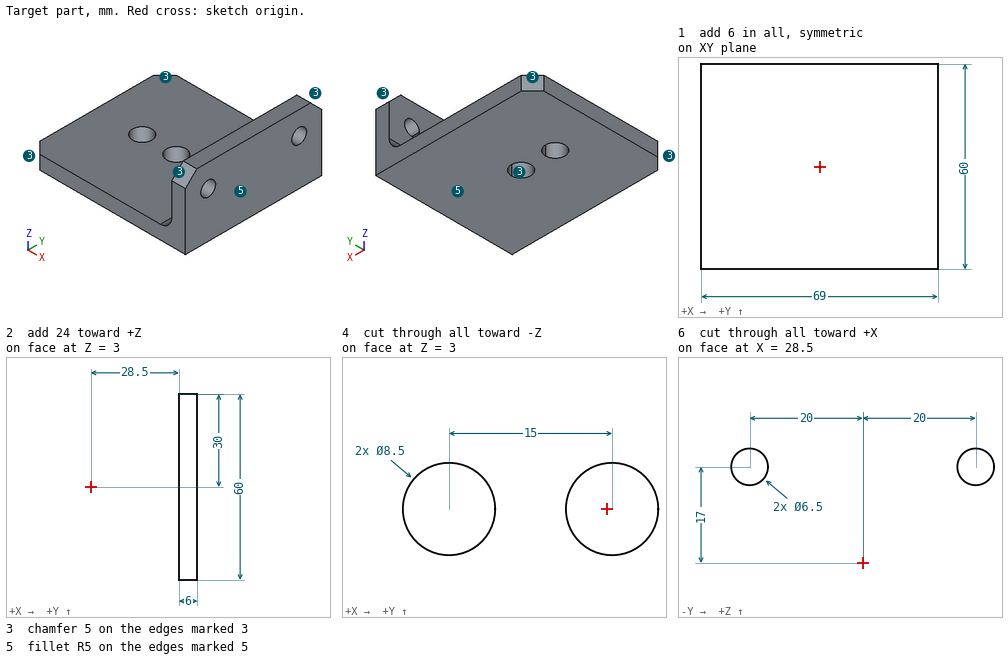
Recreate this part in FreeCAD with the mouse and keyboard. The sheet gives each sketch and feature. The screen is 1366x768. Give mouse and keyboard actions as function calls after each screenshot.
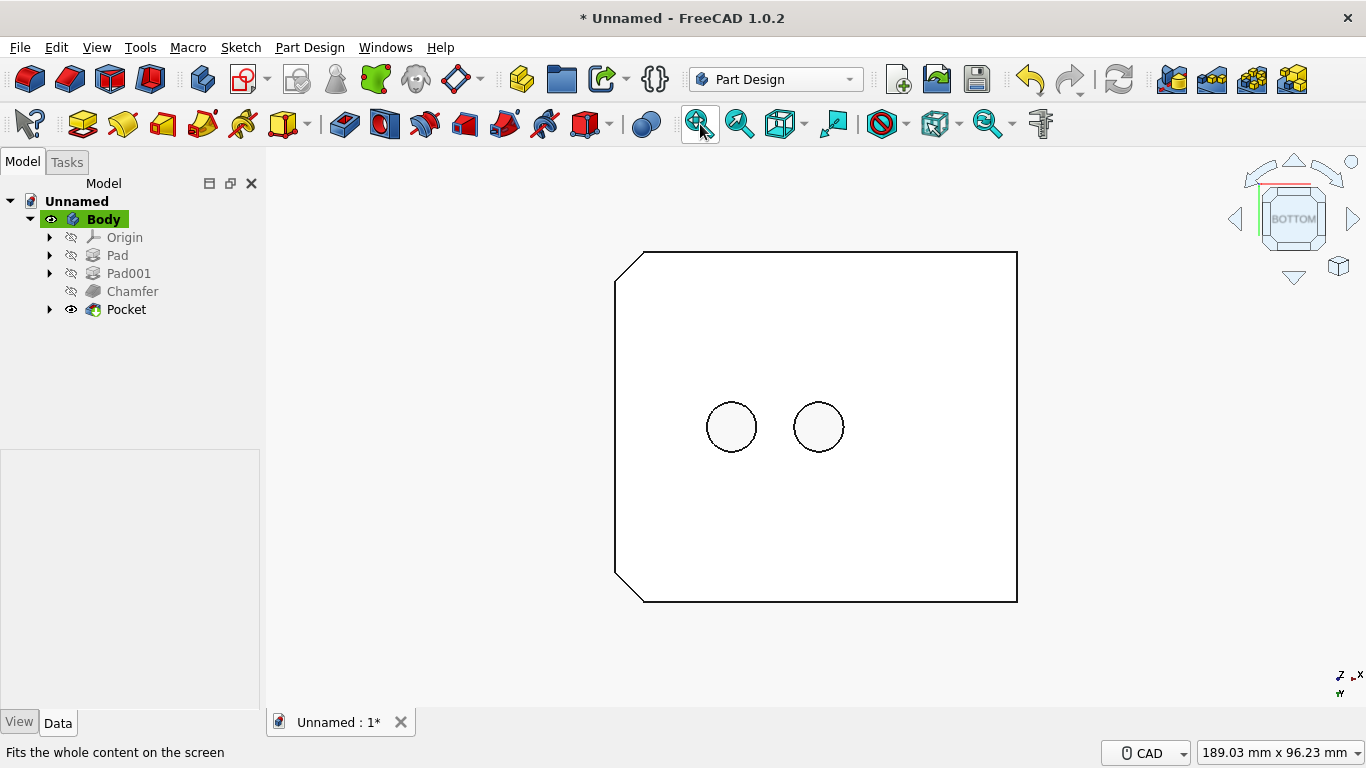
key(4)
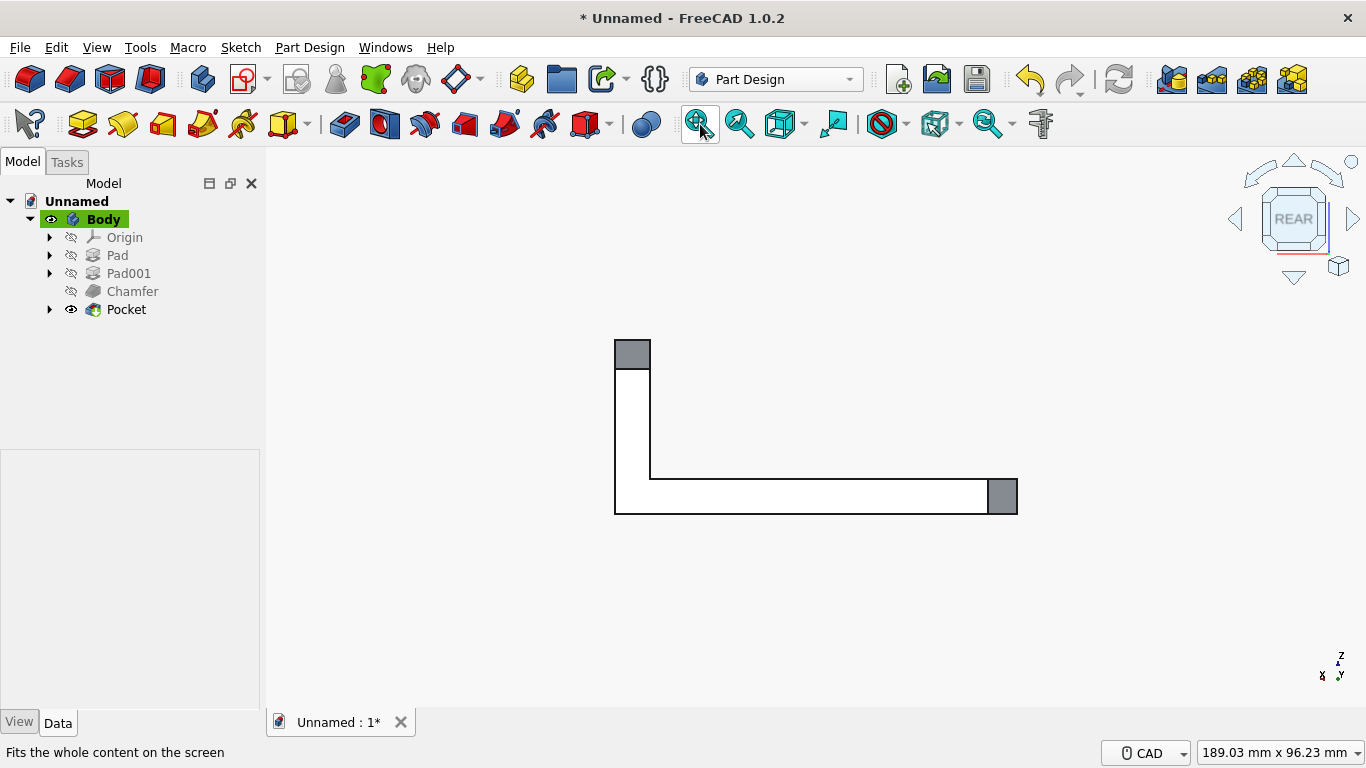
key(v)
key(f)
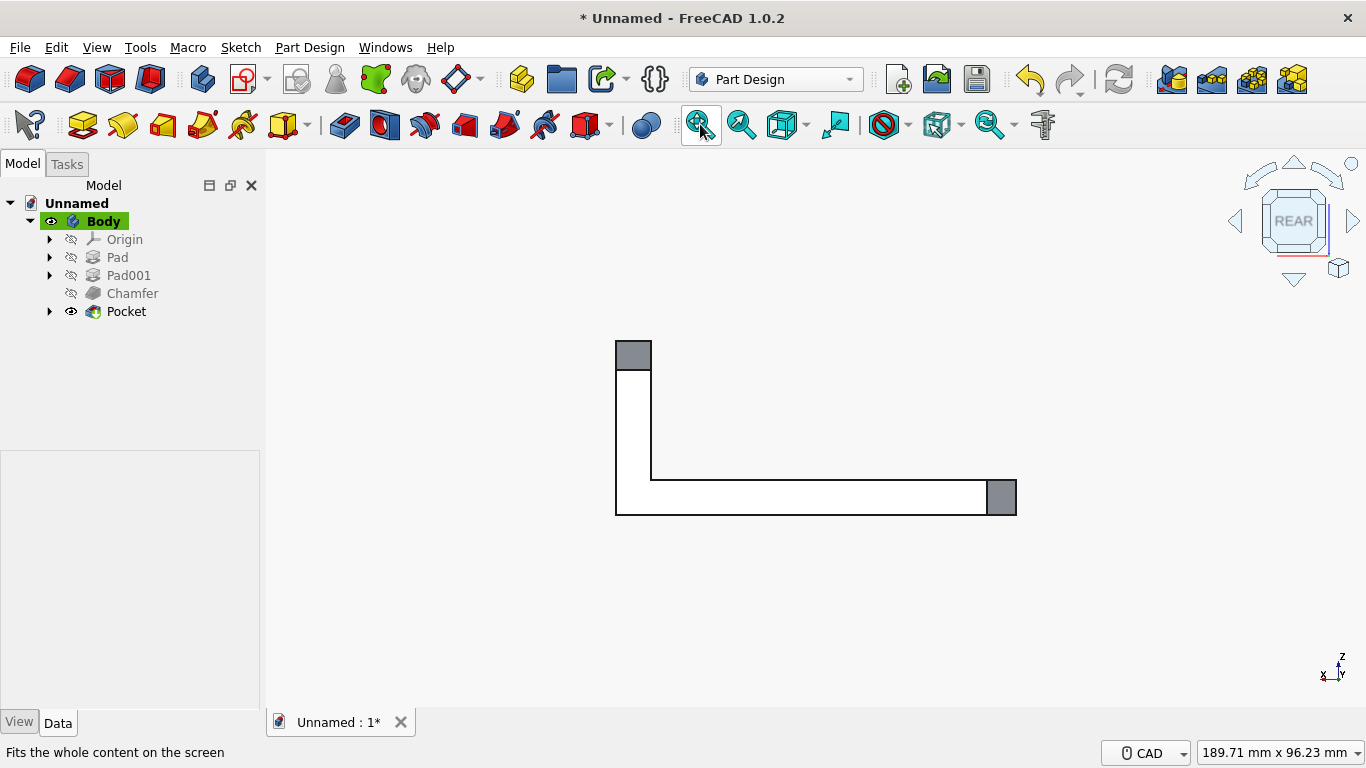
key(6)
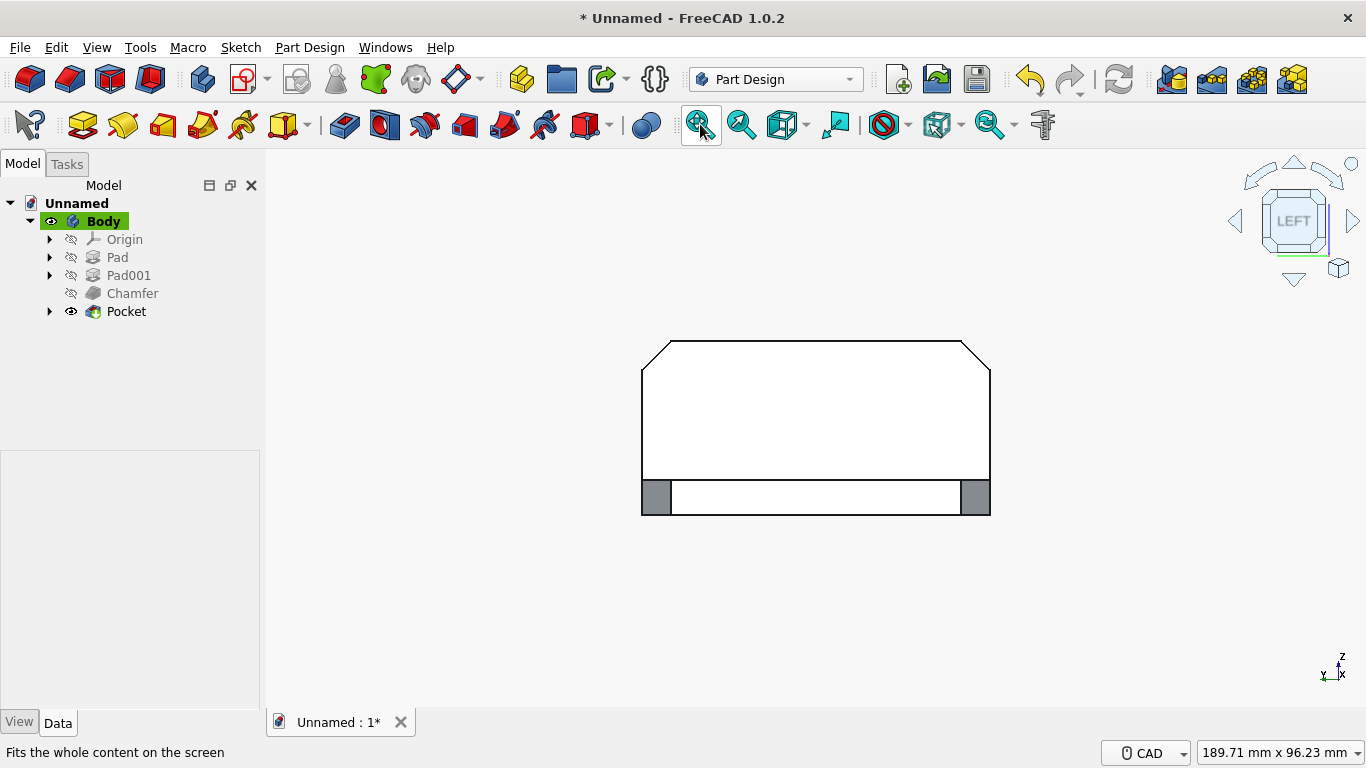
click(702, 126)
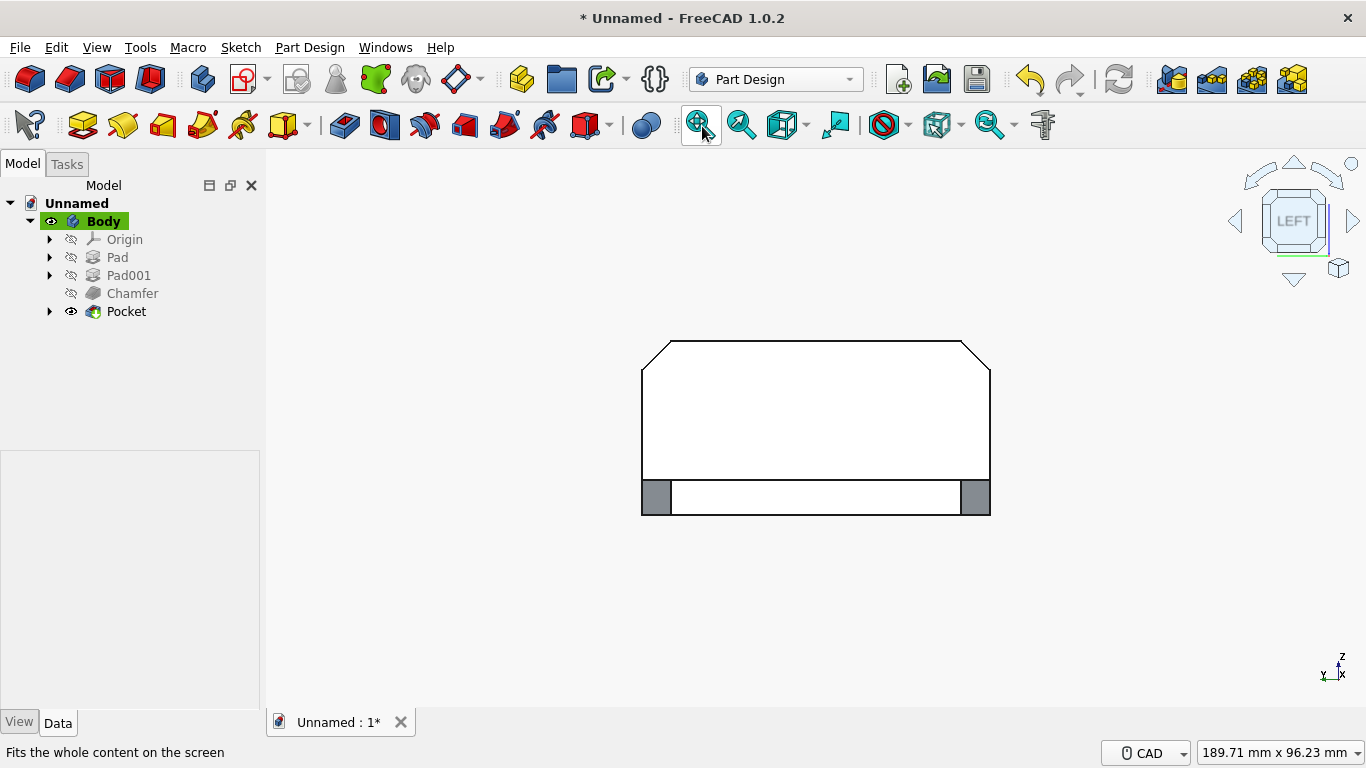
key(v)
key(3)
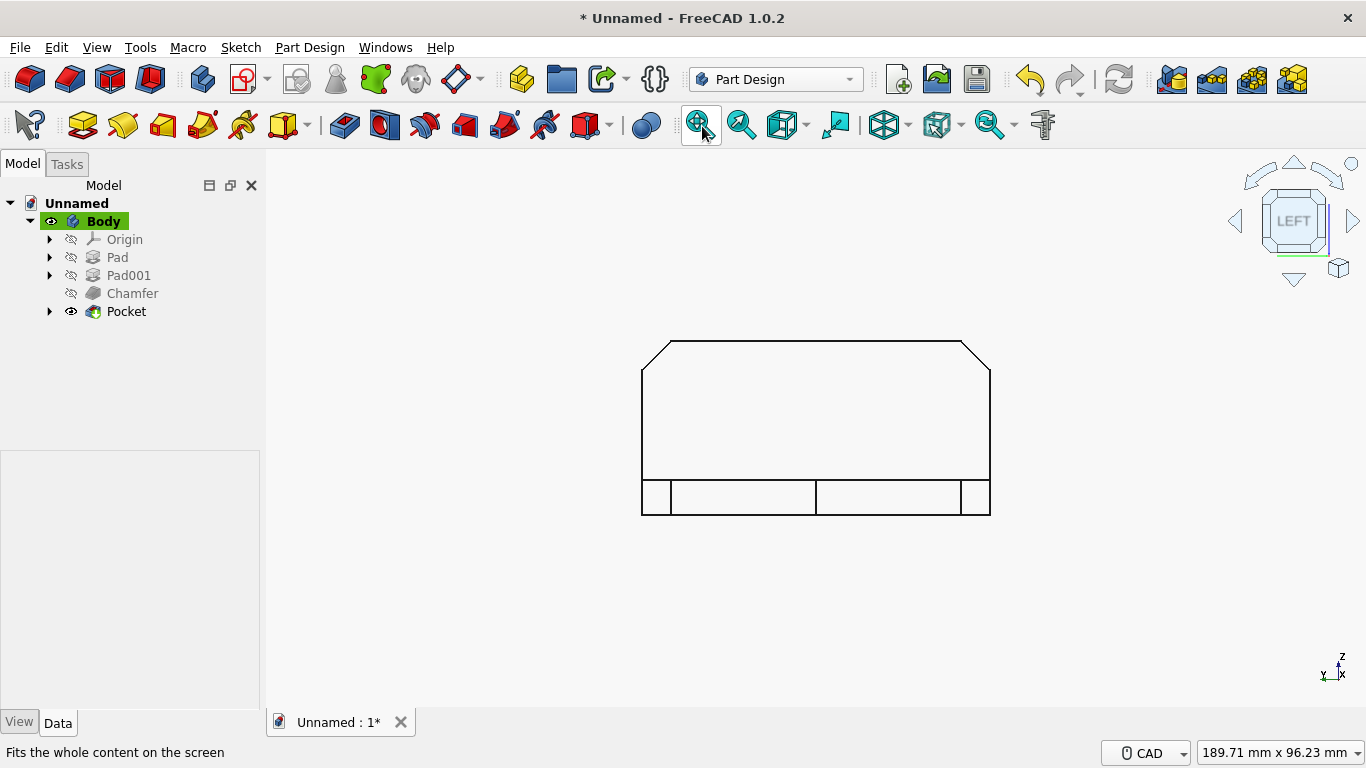
key(0)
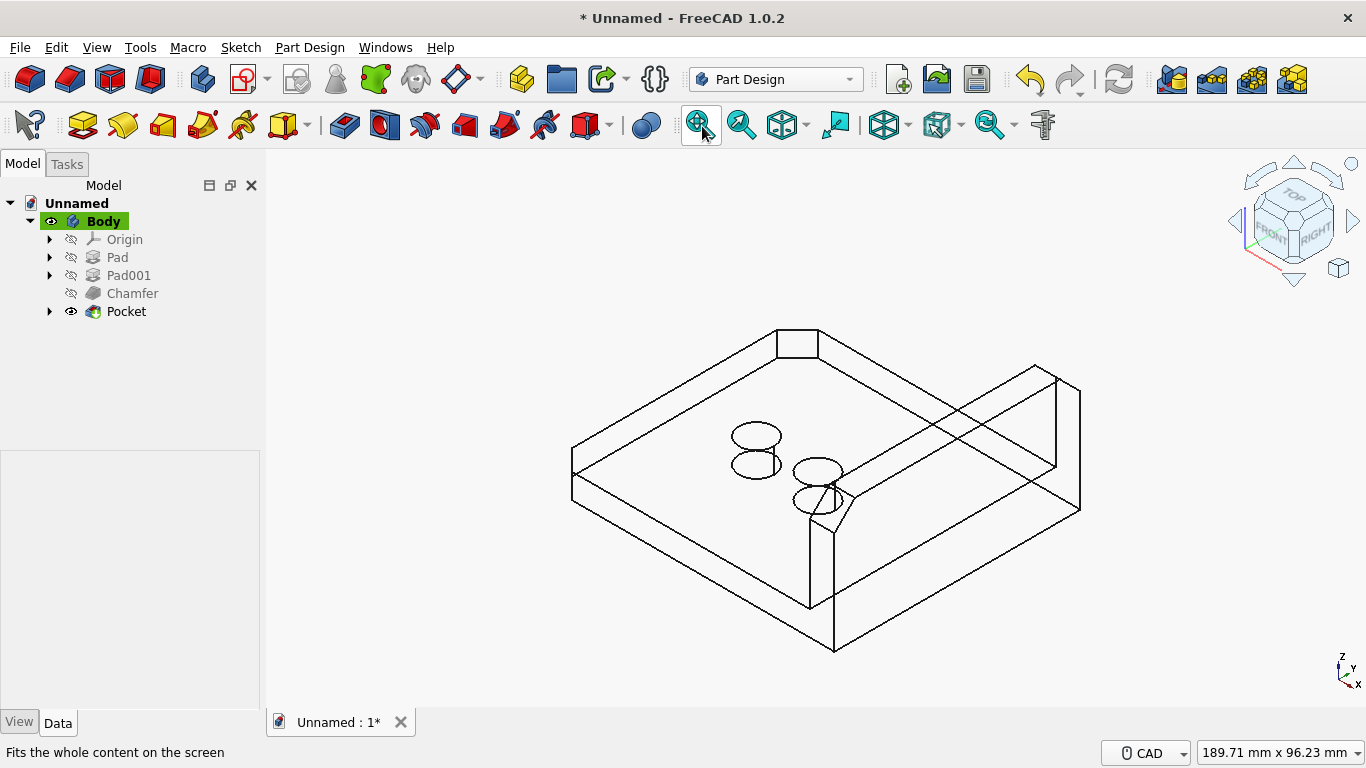
click(933, 537)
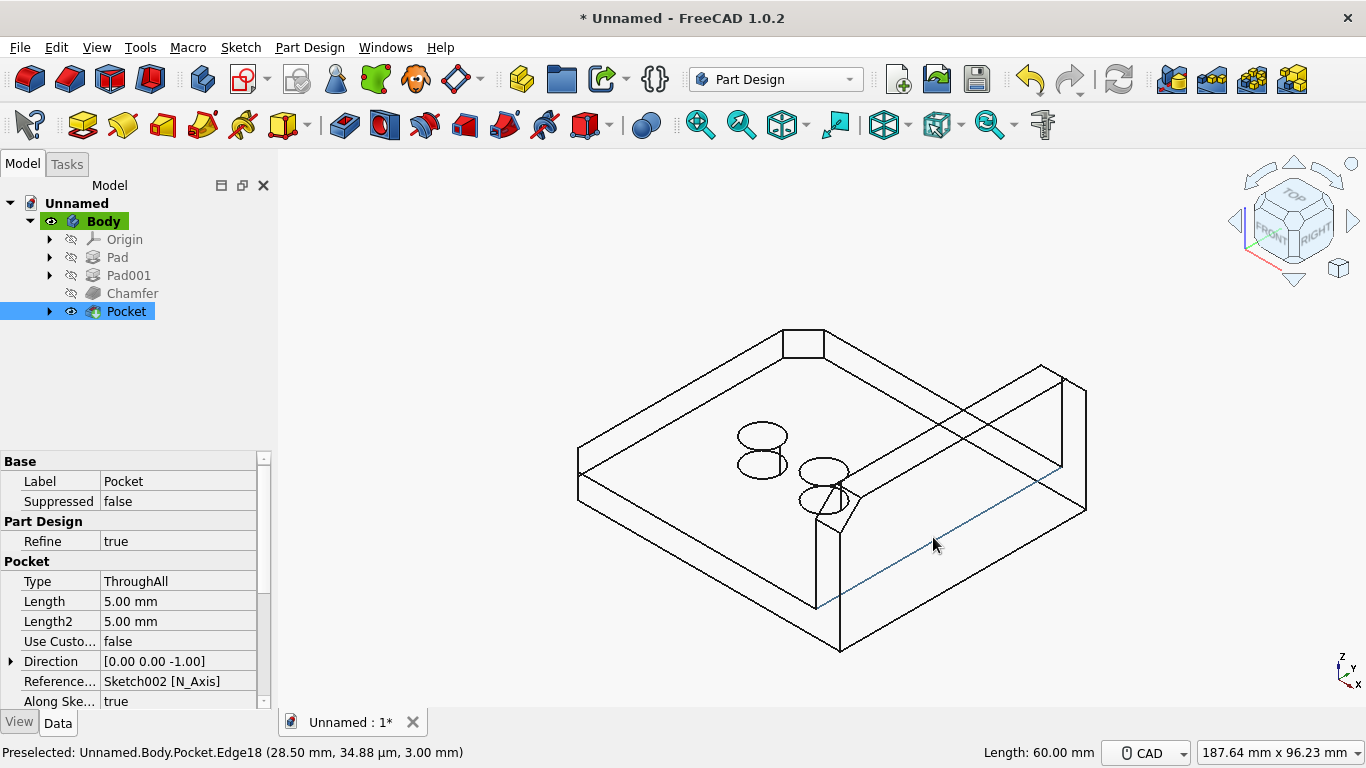
key(v)
key(1)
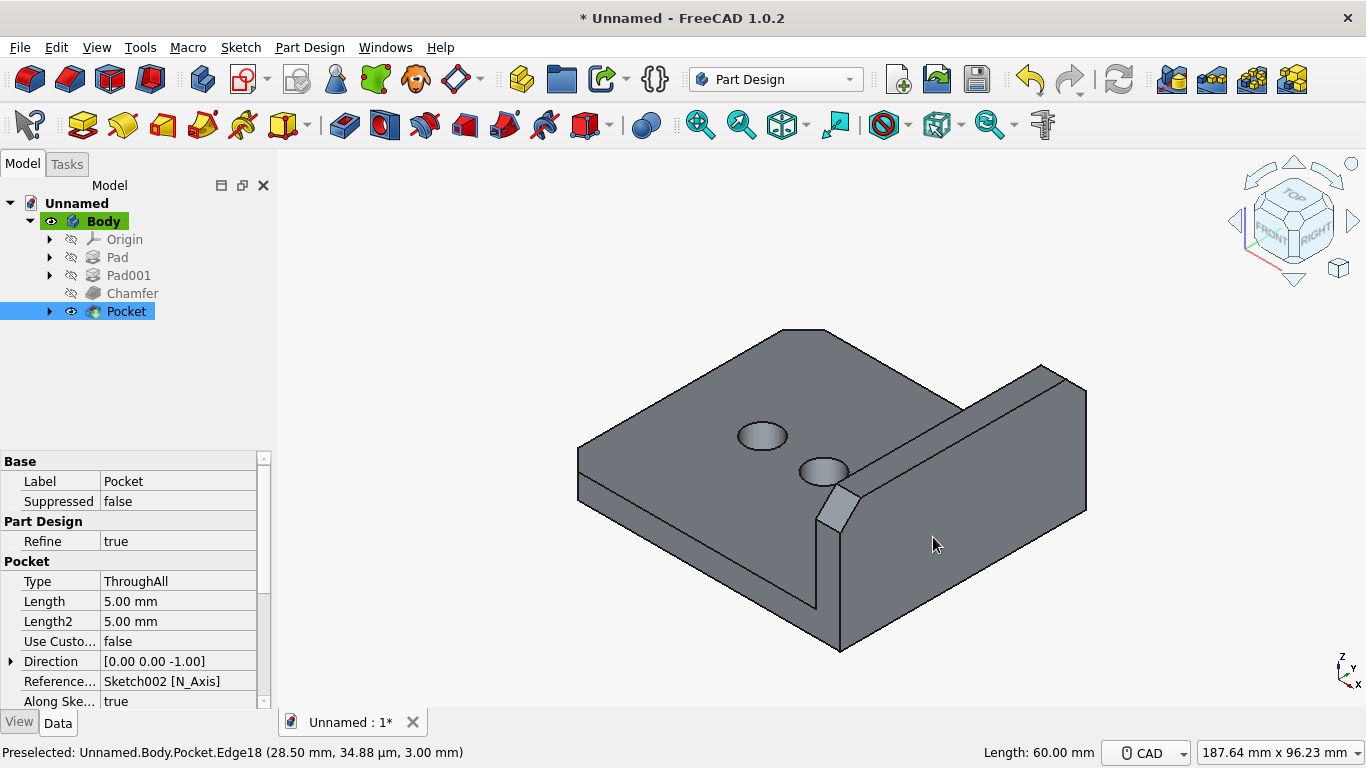
click(30, 80)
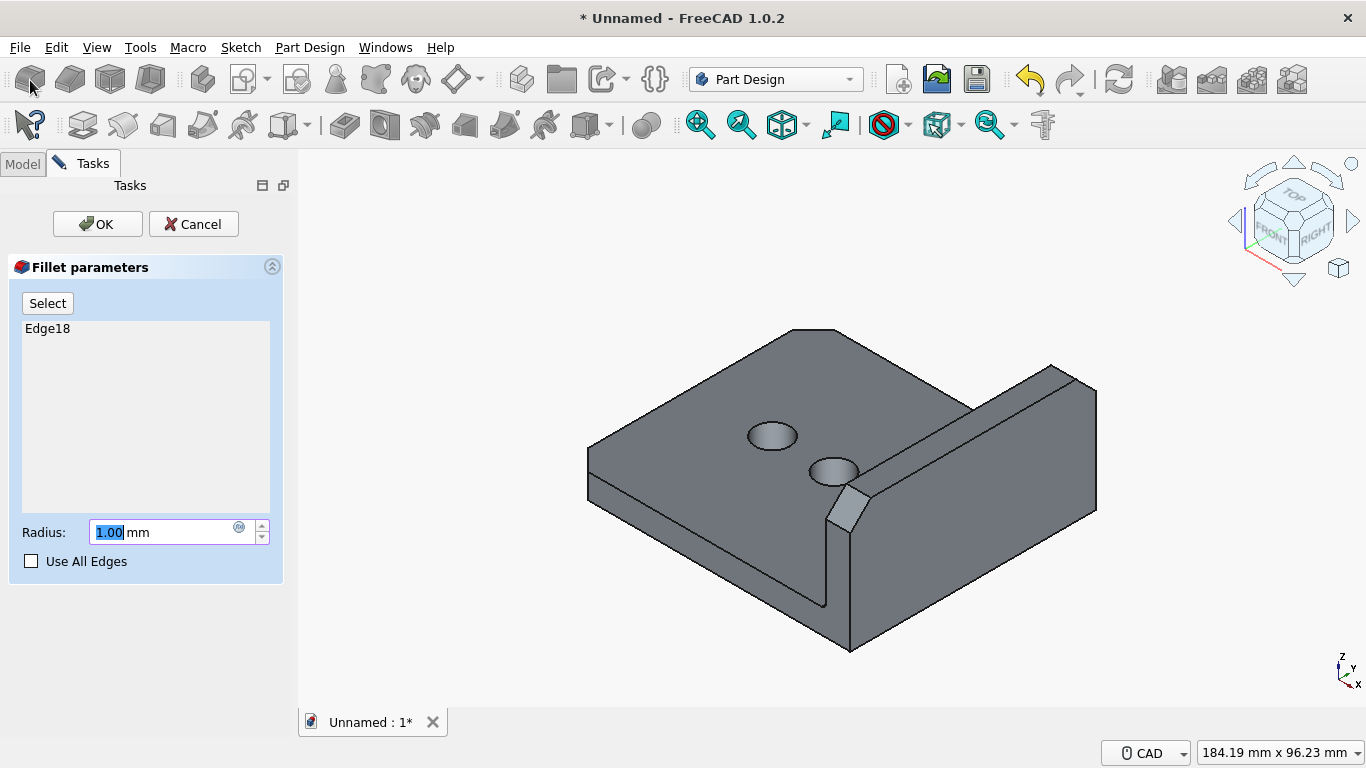
text(5)
key(Tab)